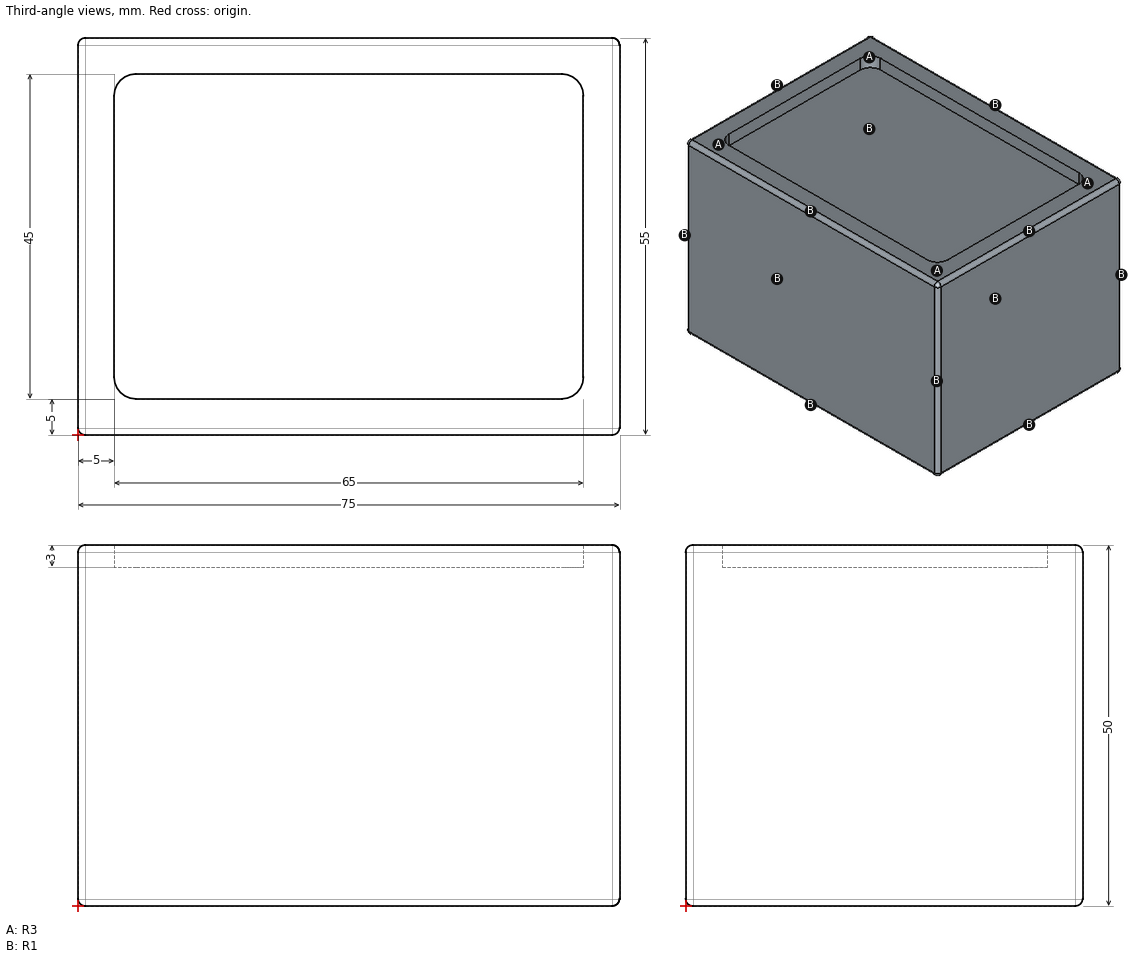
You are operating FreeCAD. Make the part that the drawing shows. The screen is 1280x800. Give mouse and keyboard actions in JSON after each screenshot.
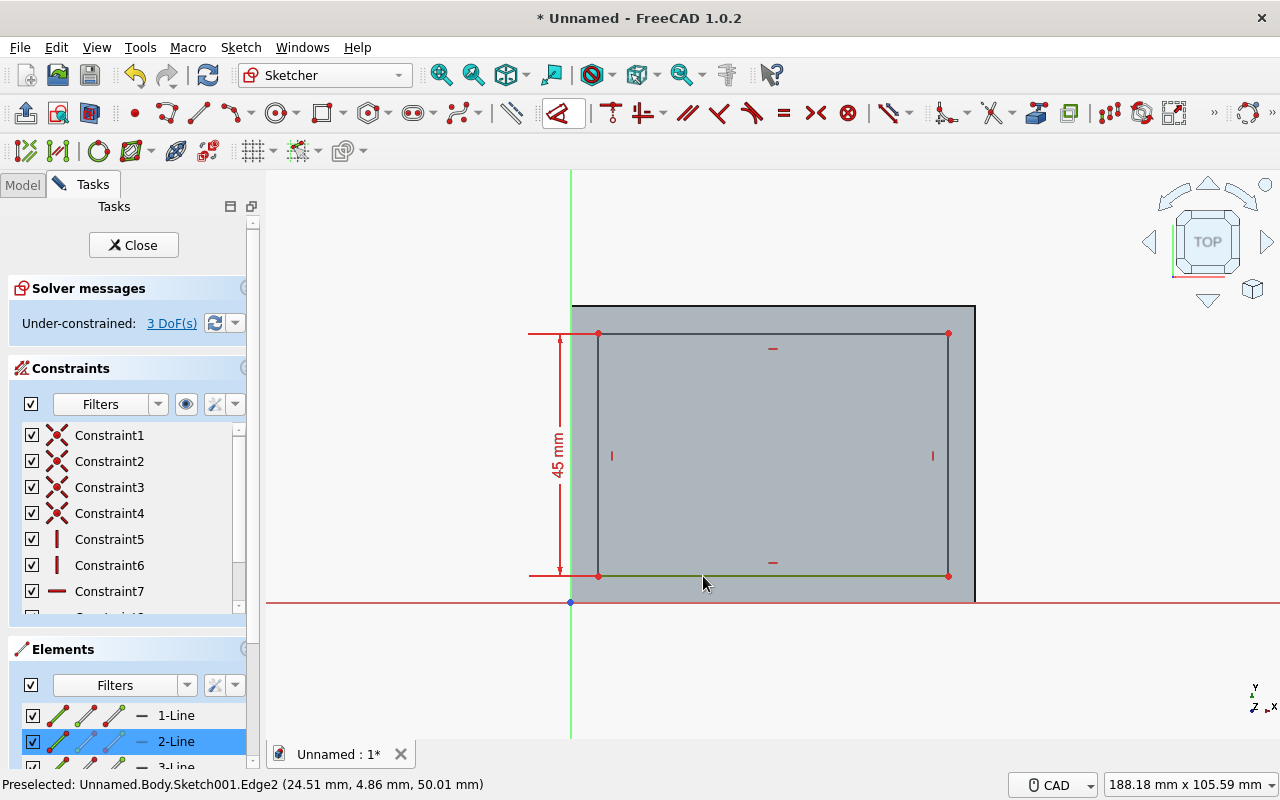
{"action": "key", "text": "l"}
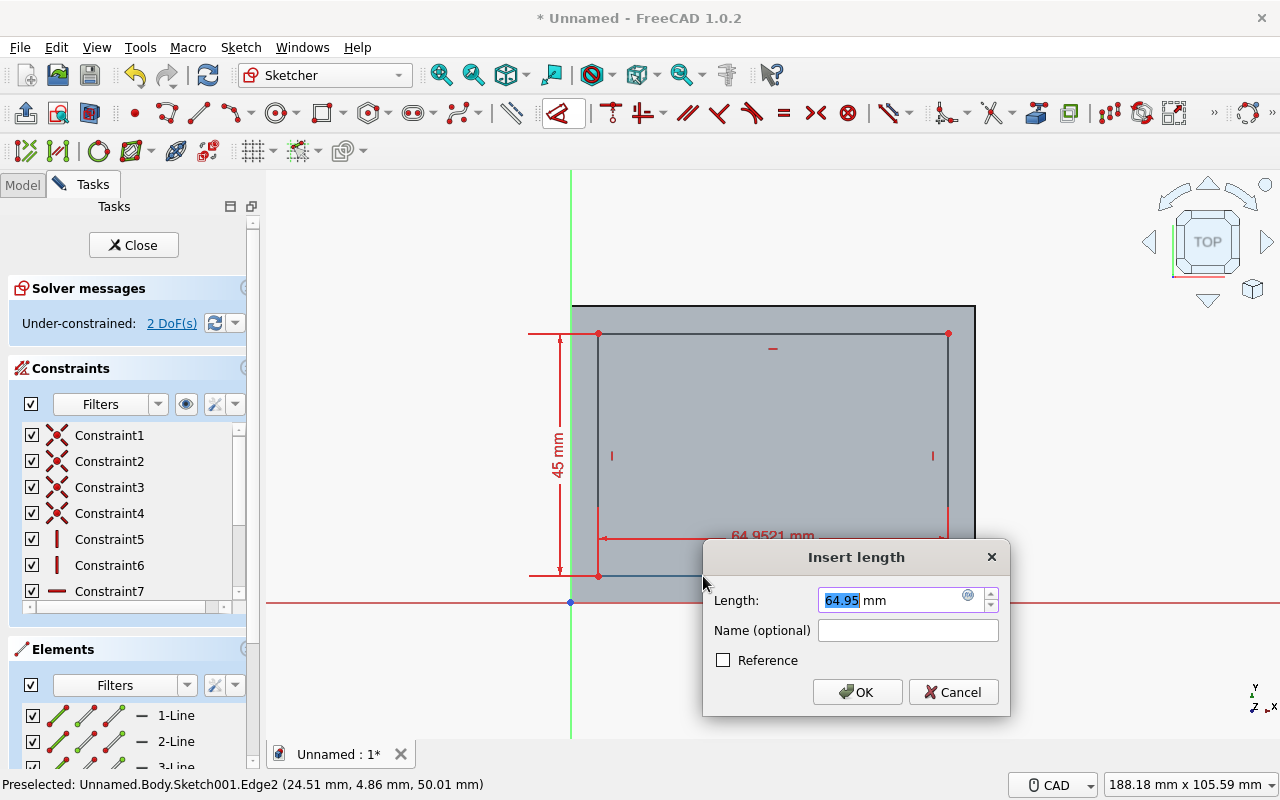
{"action": "type", "text": "65"}
{"action": "key", "text": "Return"}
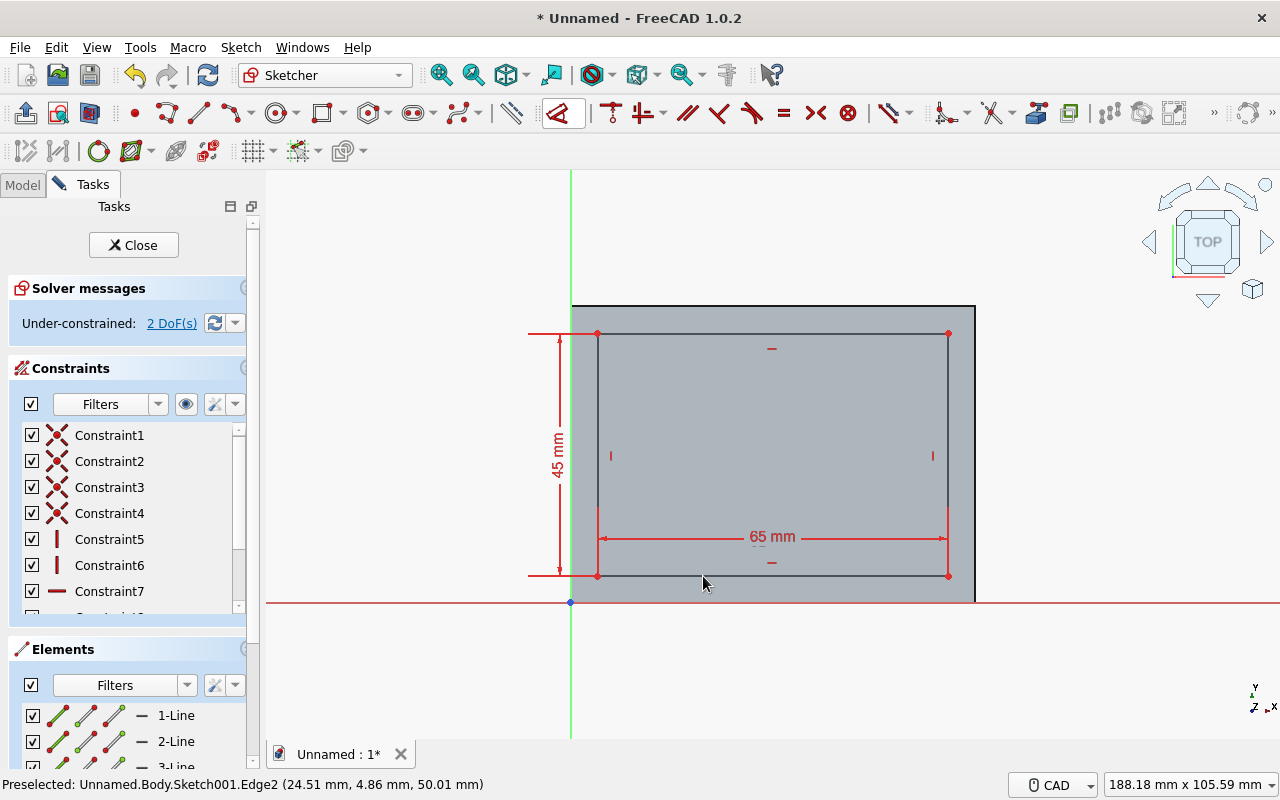
{"action": "scroll", "coordinate": [598, 334], "scroll_direction": "up", "scroll_amount": 2}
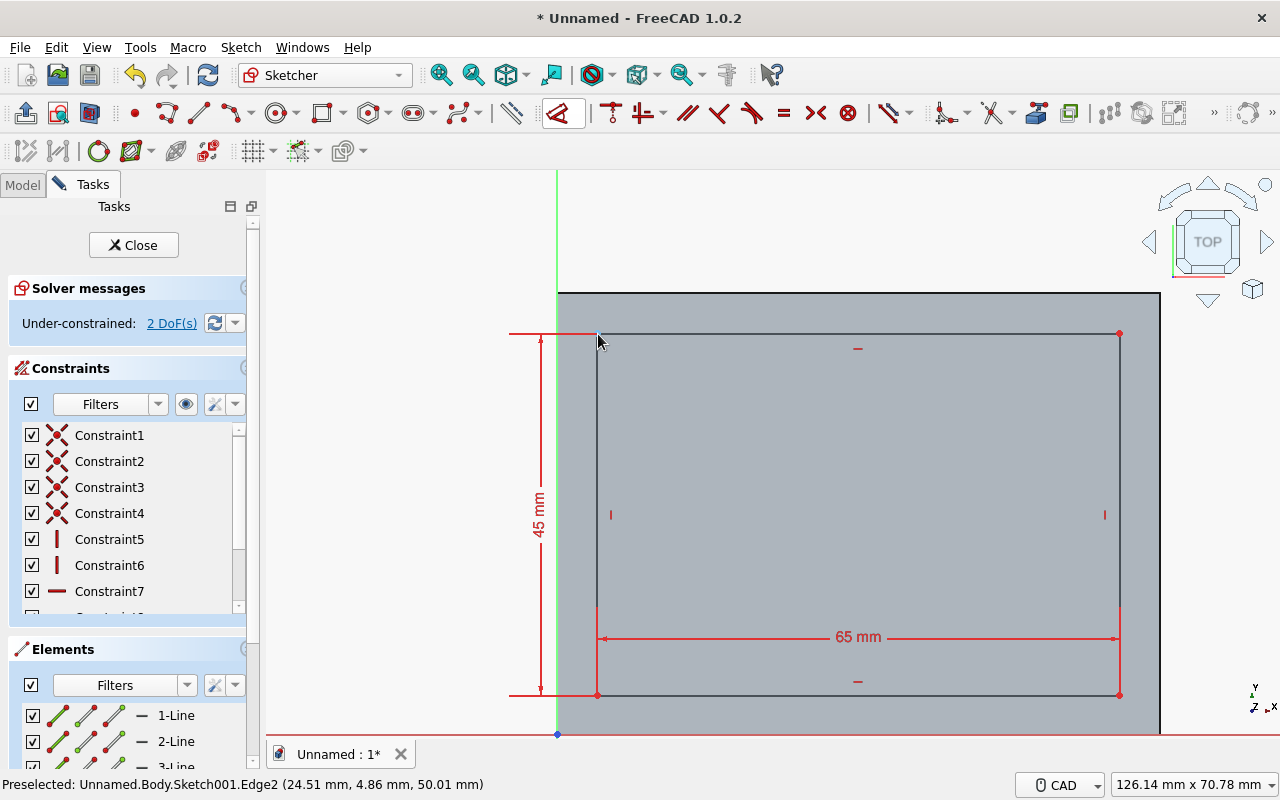
{"action": "left_click", "coordinate": [597, 334]}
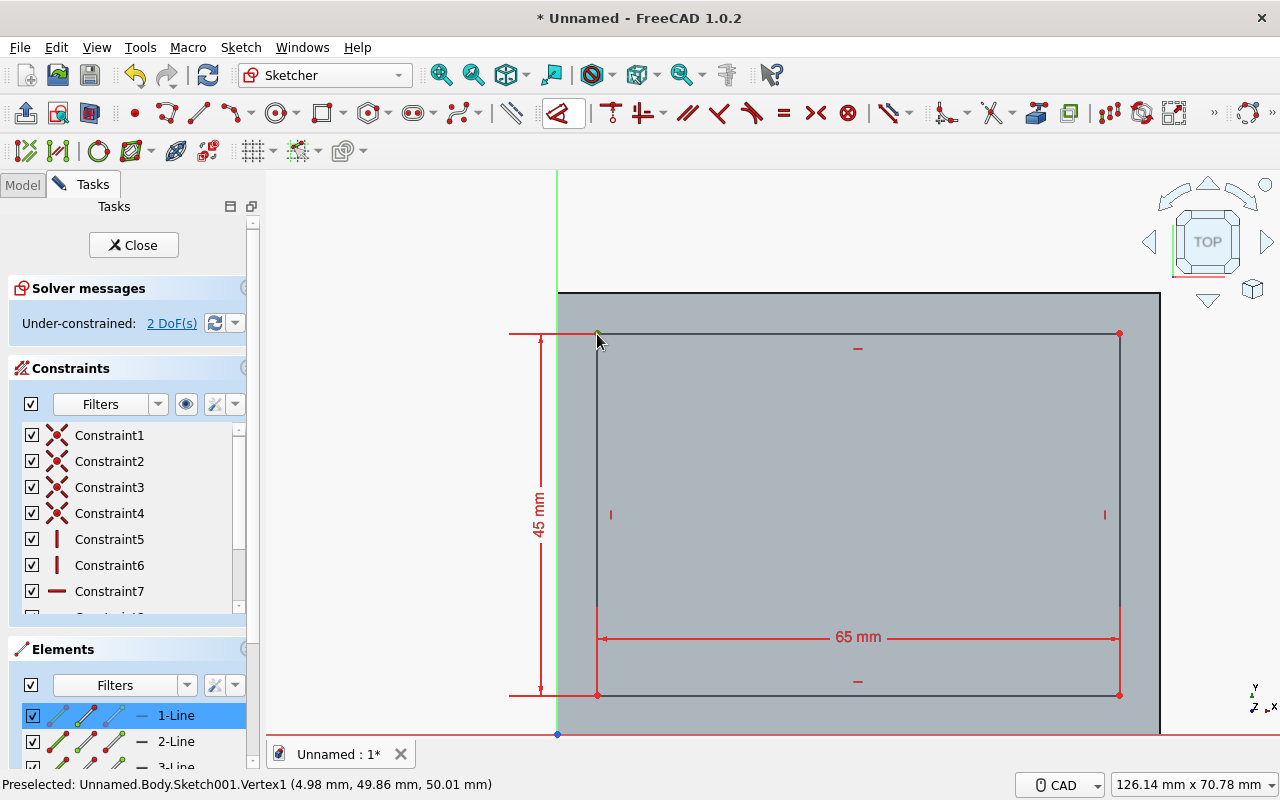
{"action": "key", "text": "l"}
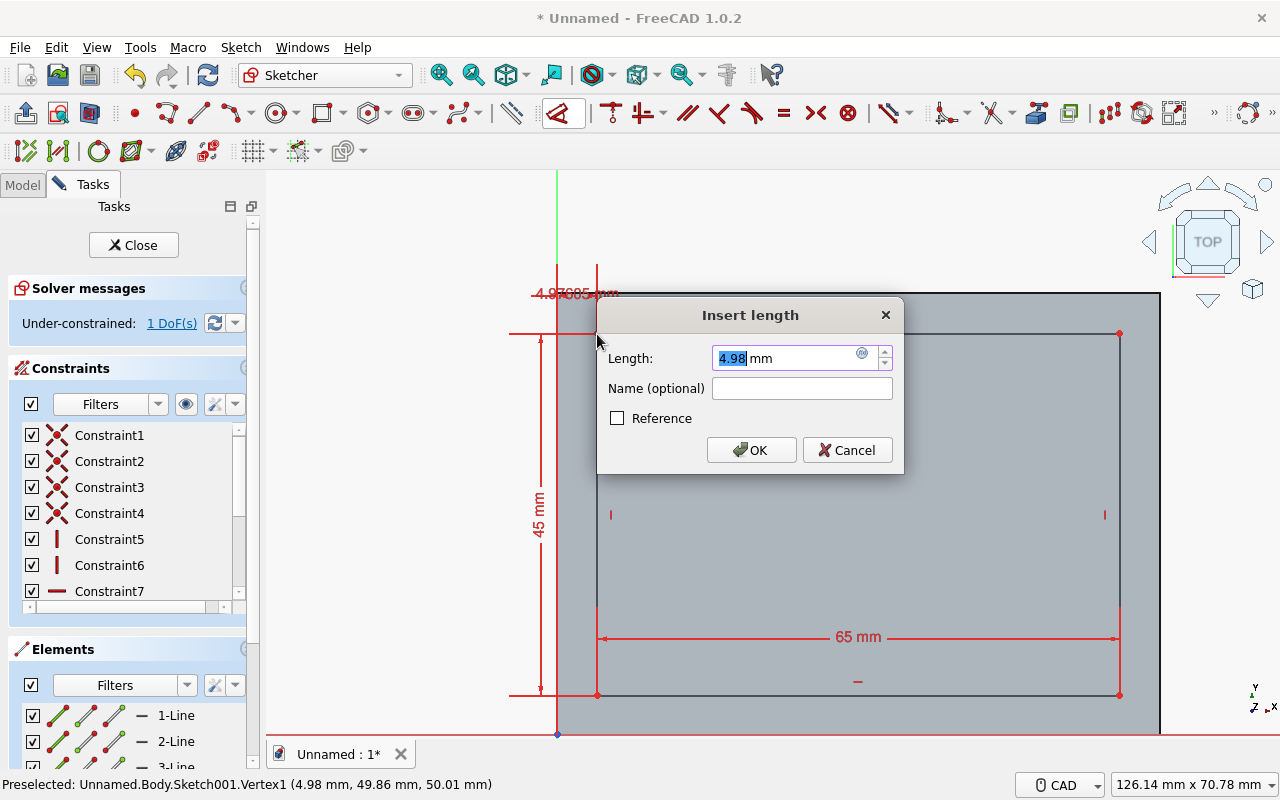
{"action": "type", "text": "5"}
{"action": "key", "text": "Return"}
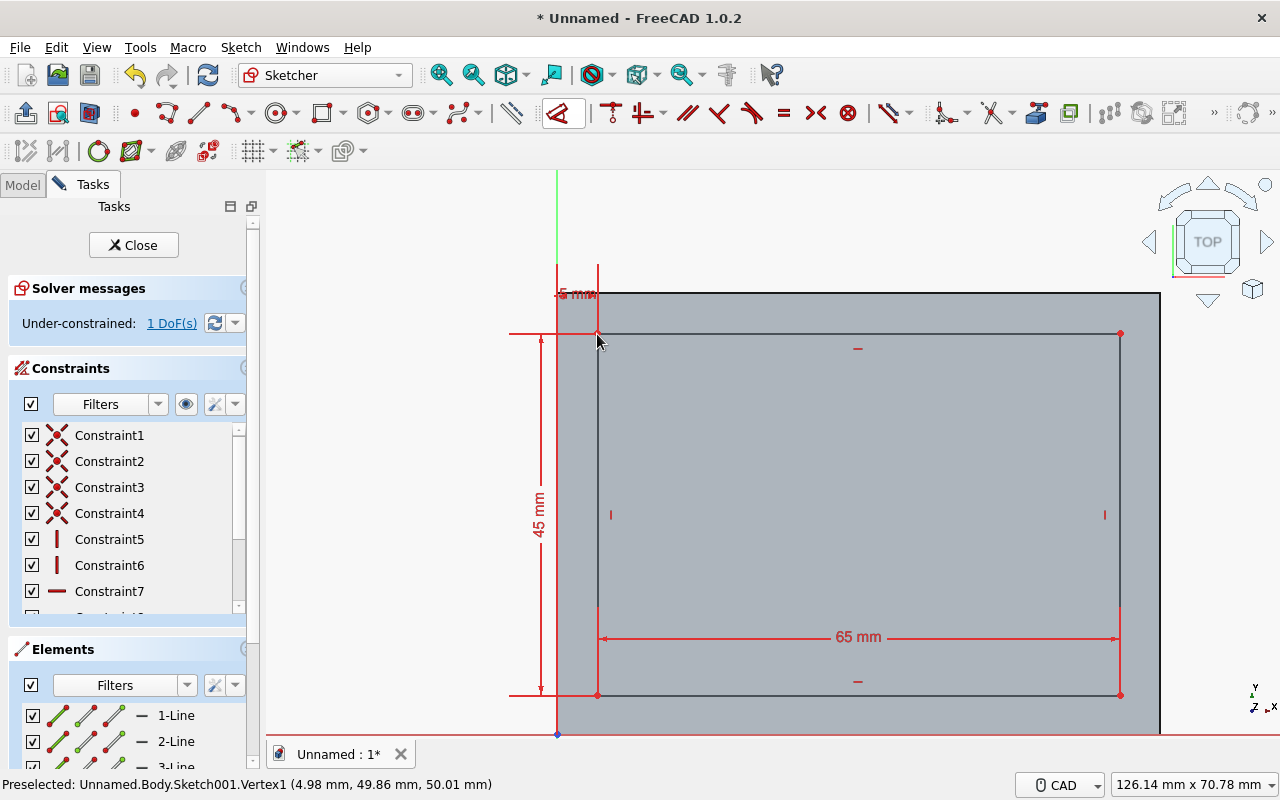
{"action": "left_click", "coordinate": [598, 696]}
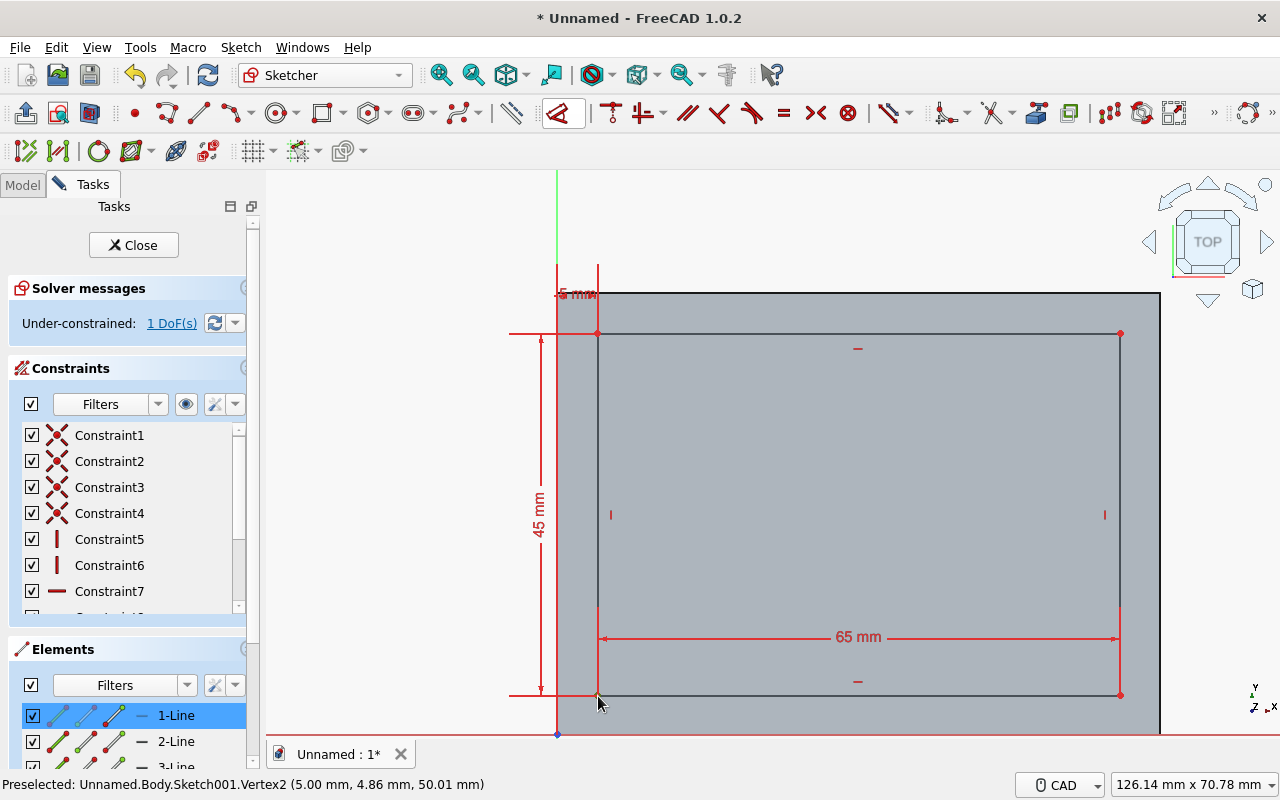
{"action": "key", "text": "i"}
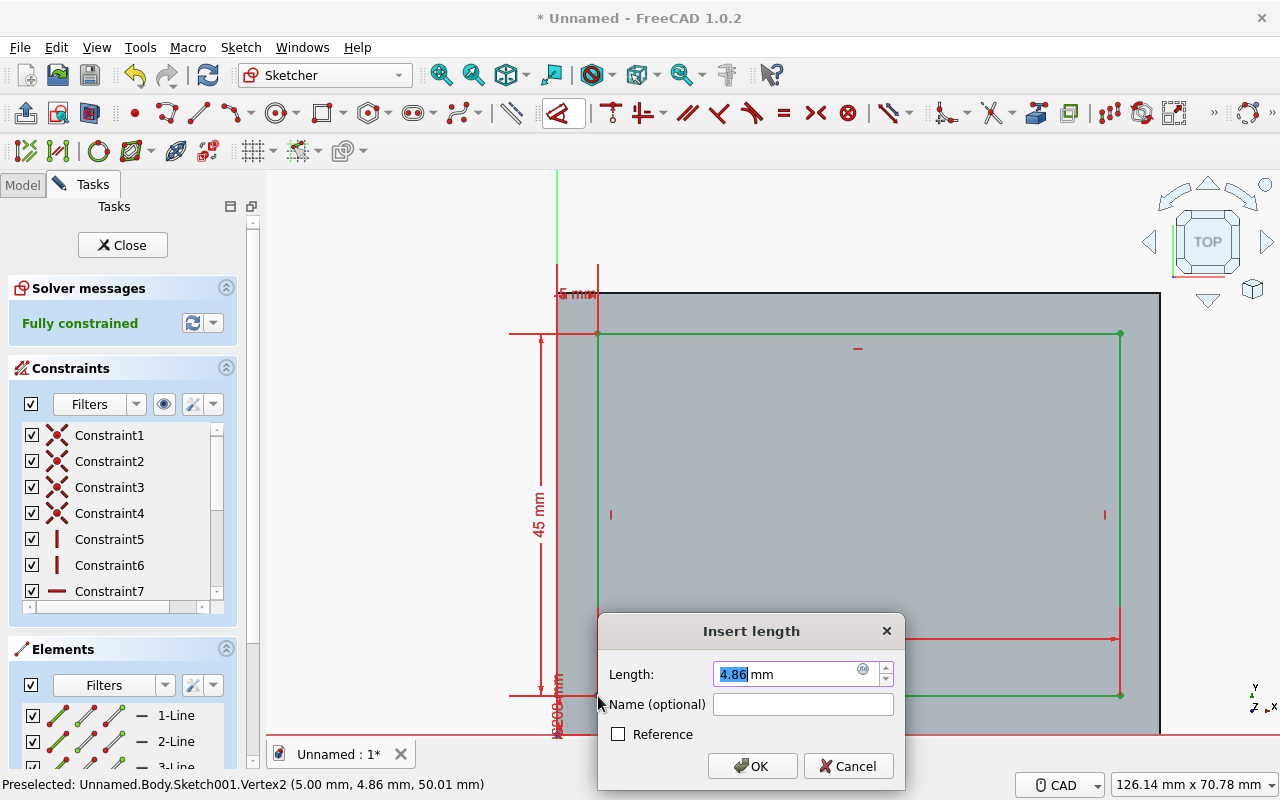
{"action": "type", "text": "5"}
{"action": "key", "text": "Return"}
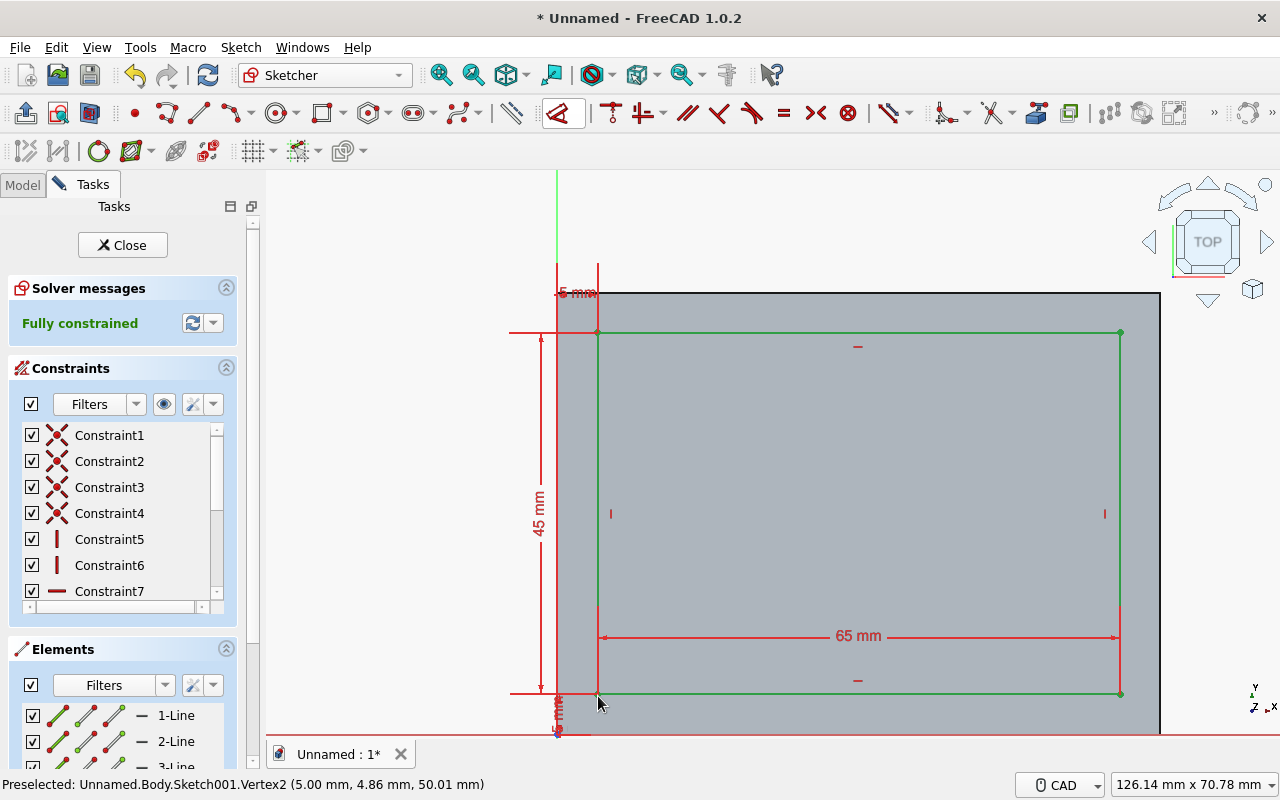
{"action": "left_click", "coordinate": [123, 245]}